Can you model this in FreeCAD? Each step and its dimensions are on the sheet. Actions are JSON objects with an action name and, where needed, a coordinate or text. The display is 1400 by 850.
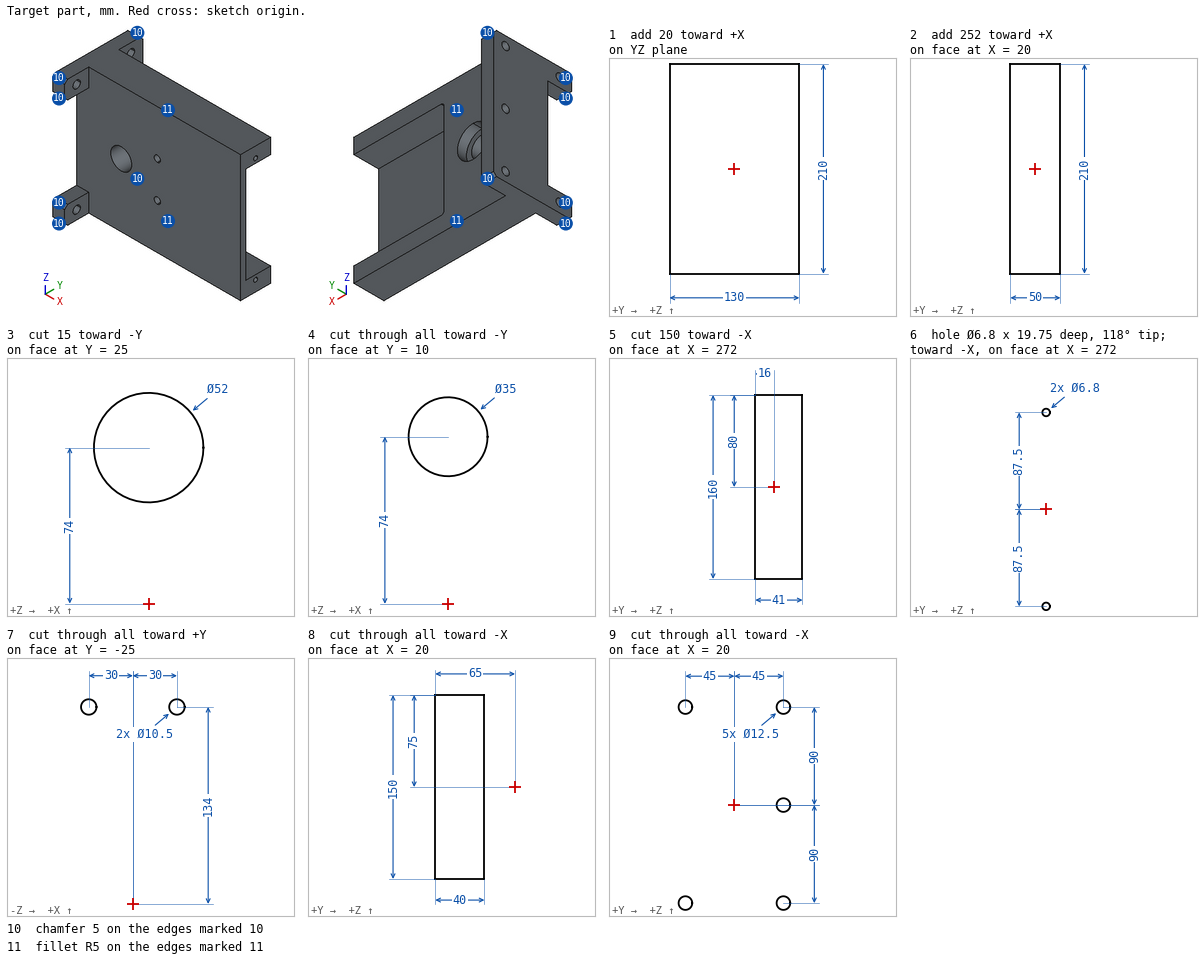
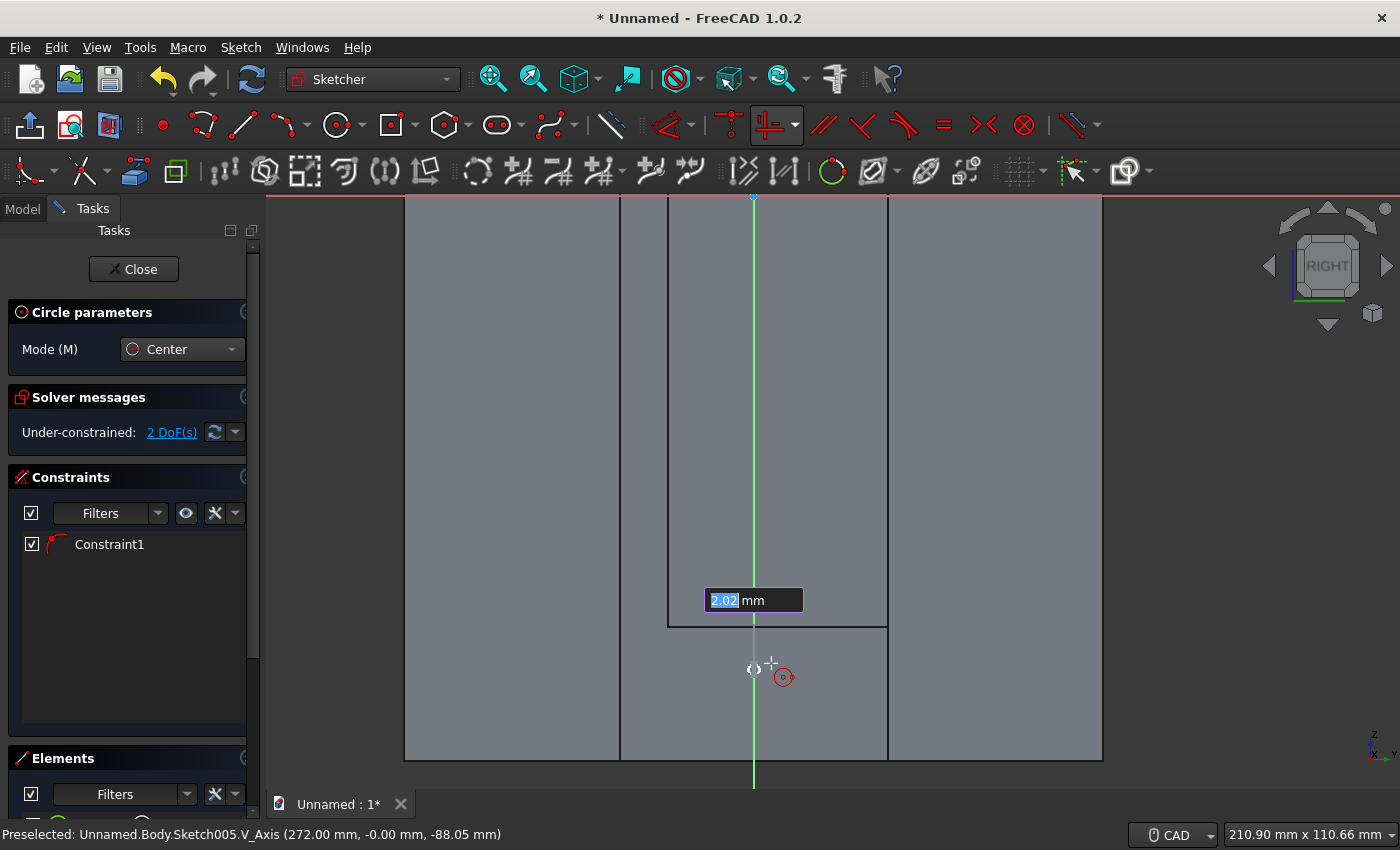
{"action": "left_click", "coordinate": [771, 661]}
{"action": "key", "text": "Escape"}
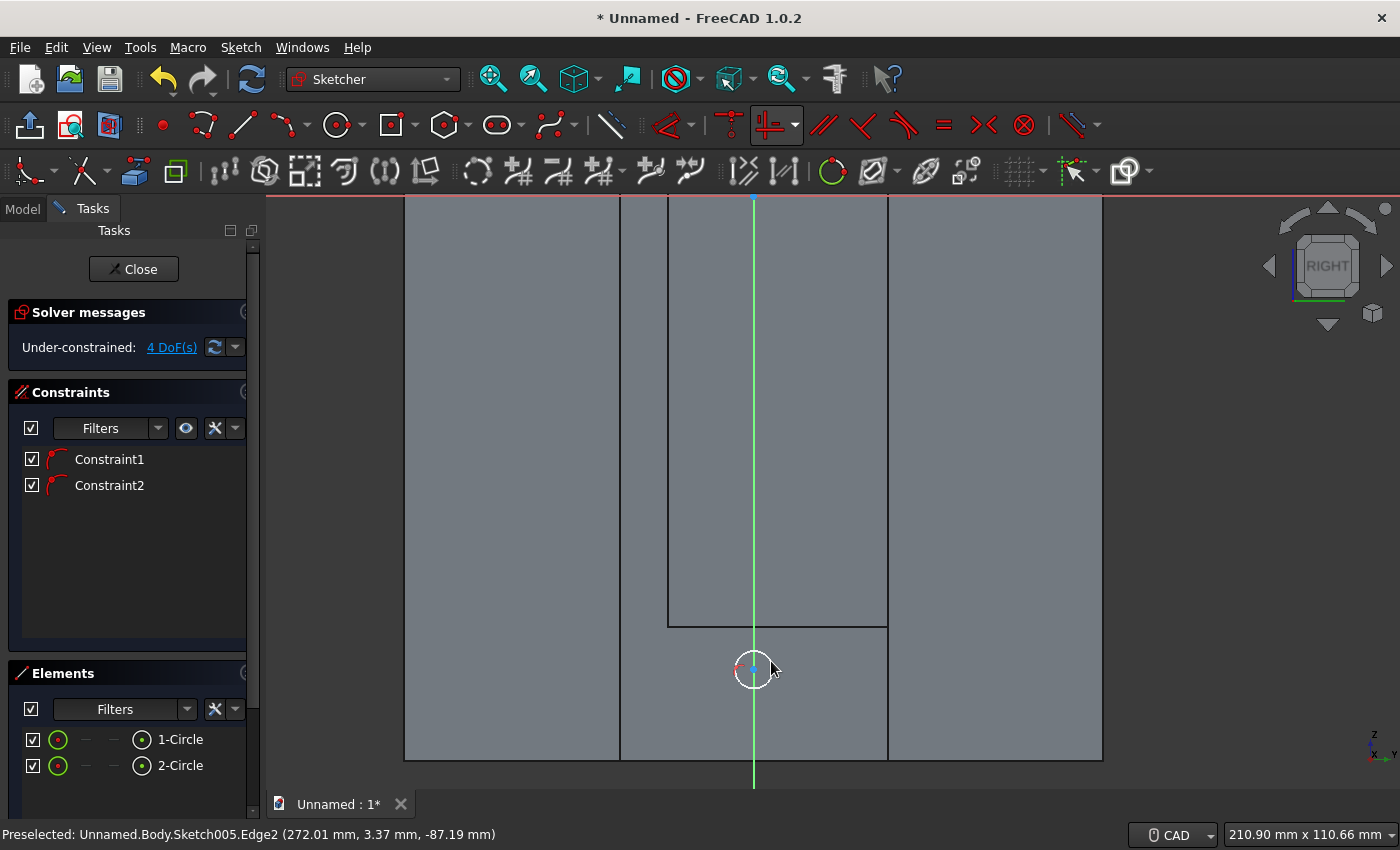
{"action": "scroll", "coordinate": [771, 663], "scroll_direction": "down", "scroll_amount": 5}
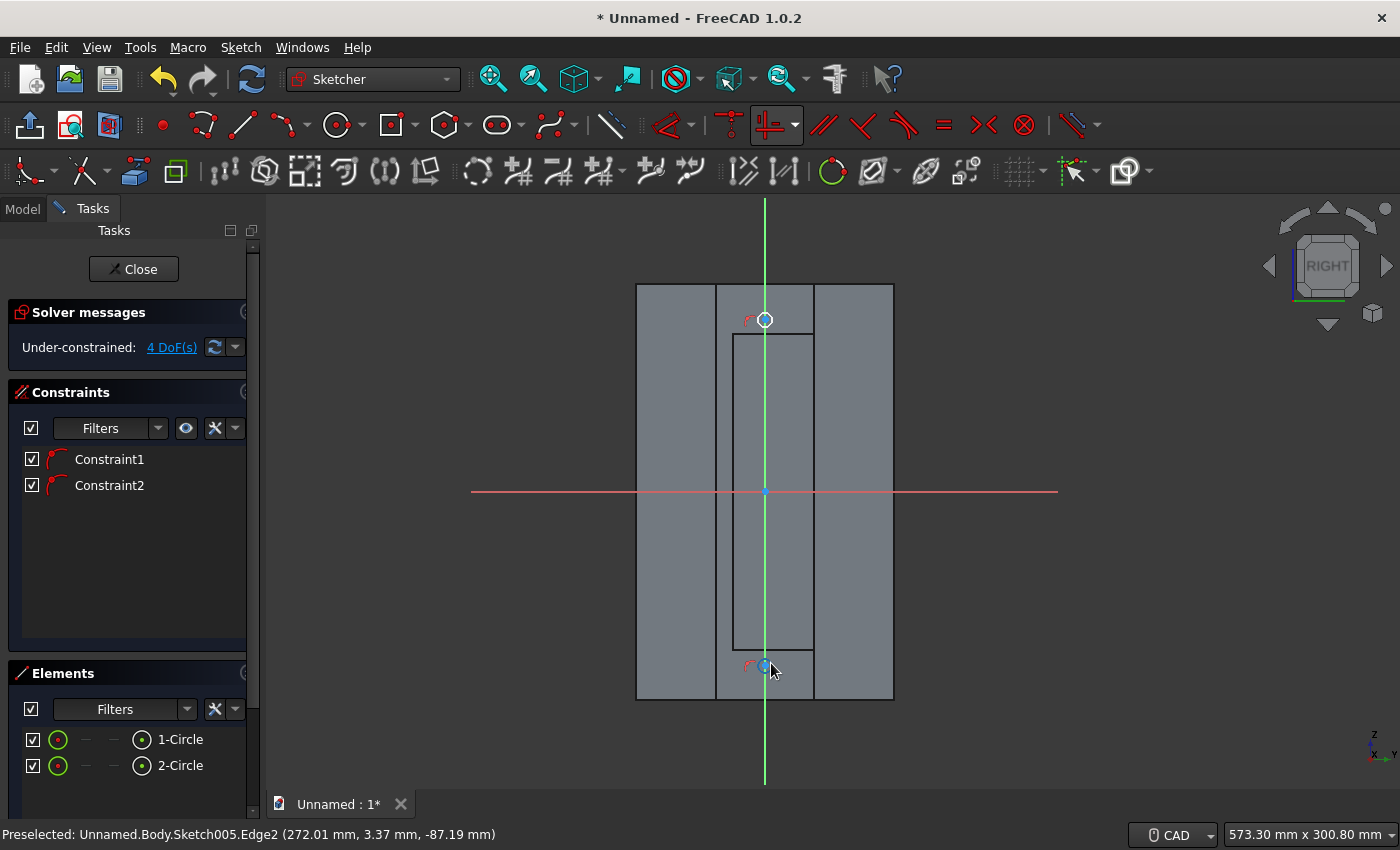
{"action": "scroll", "coordinate": [770, 315], "scroll_direction": "up", "scroll_amount": 6}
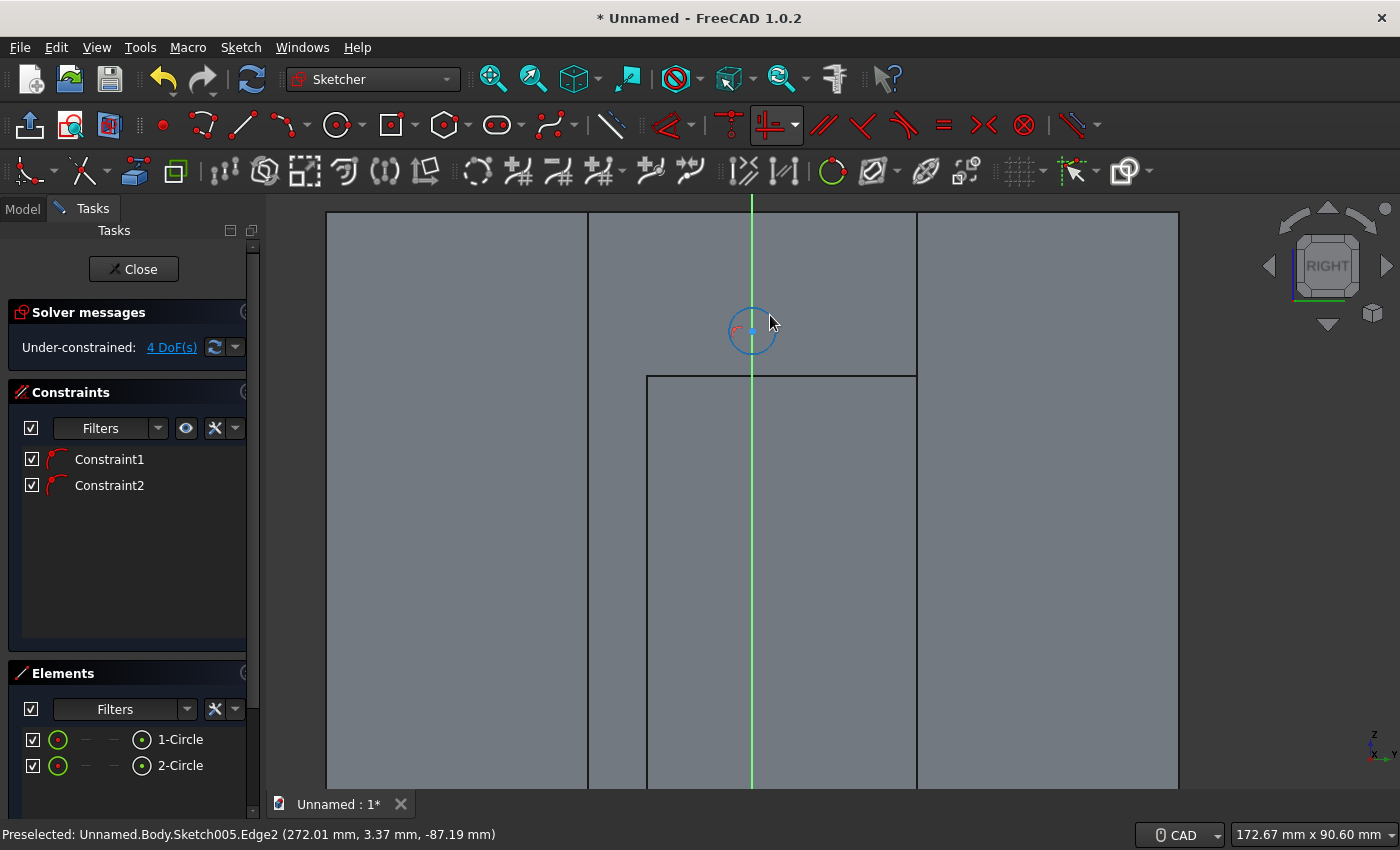
{"action": "left_click", "coordinate": [769, 315]}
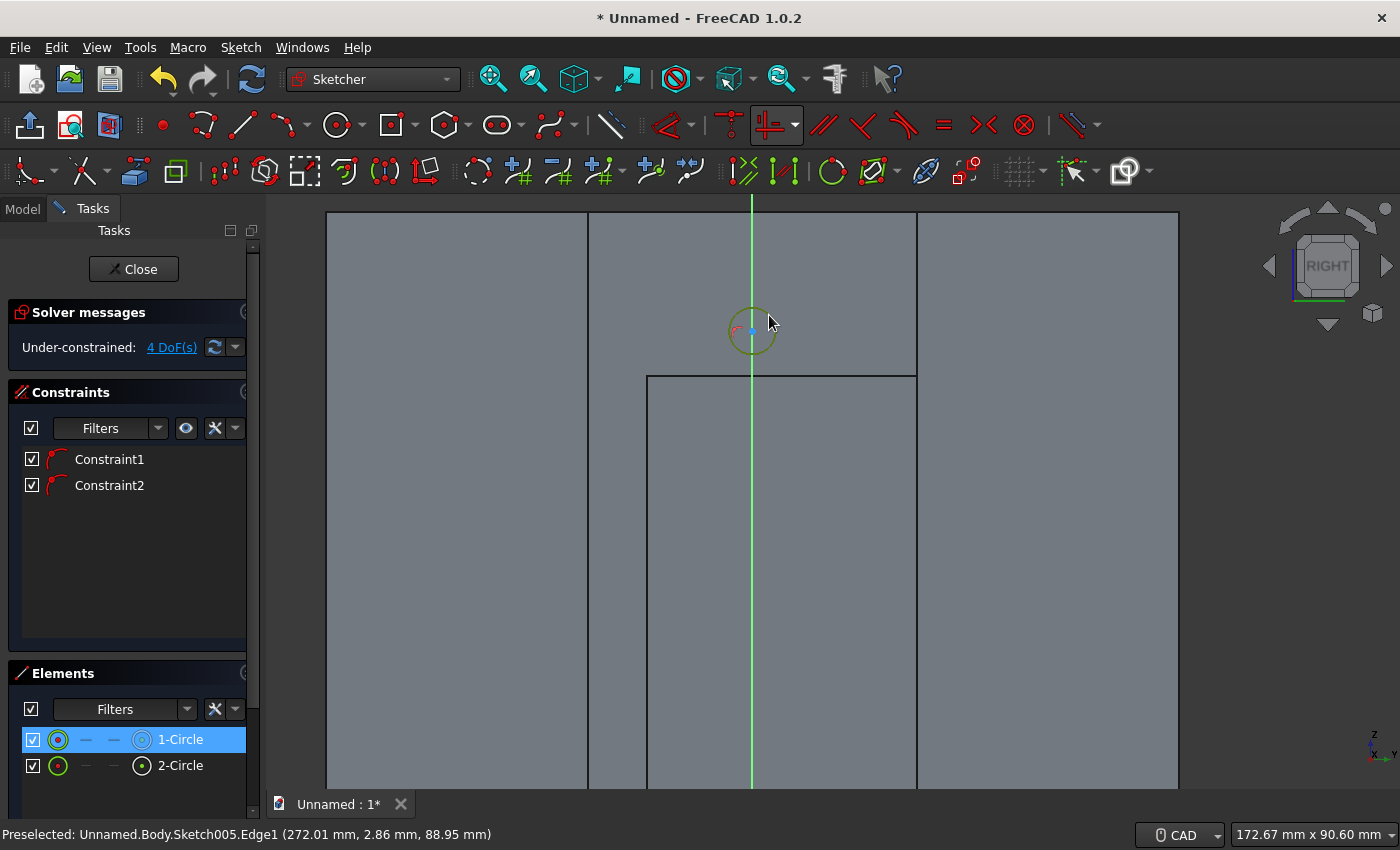
{"action": "scroll", "coordinate": [770, 315], "scroll_direction": "down", "scroll_amount": 6}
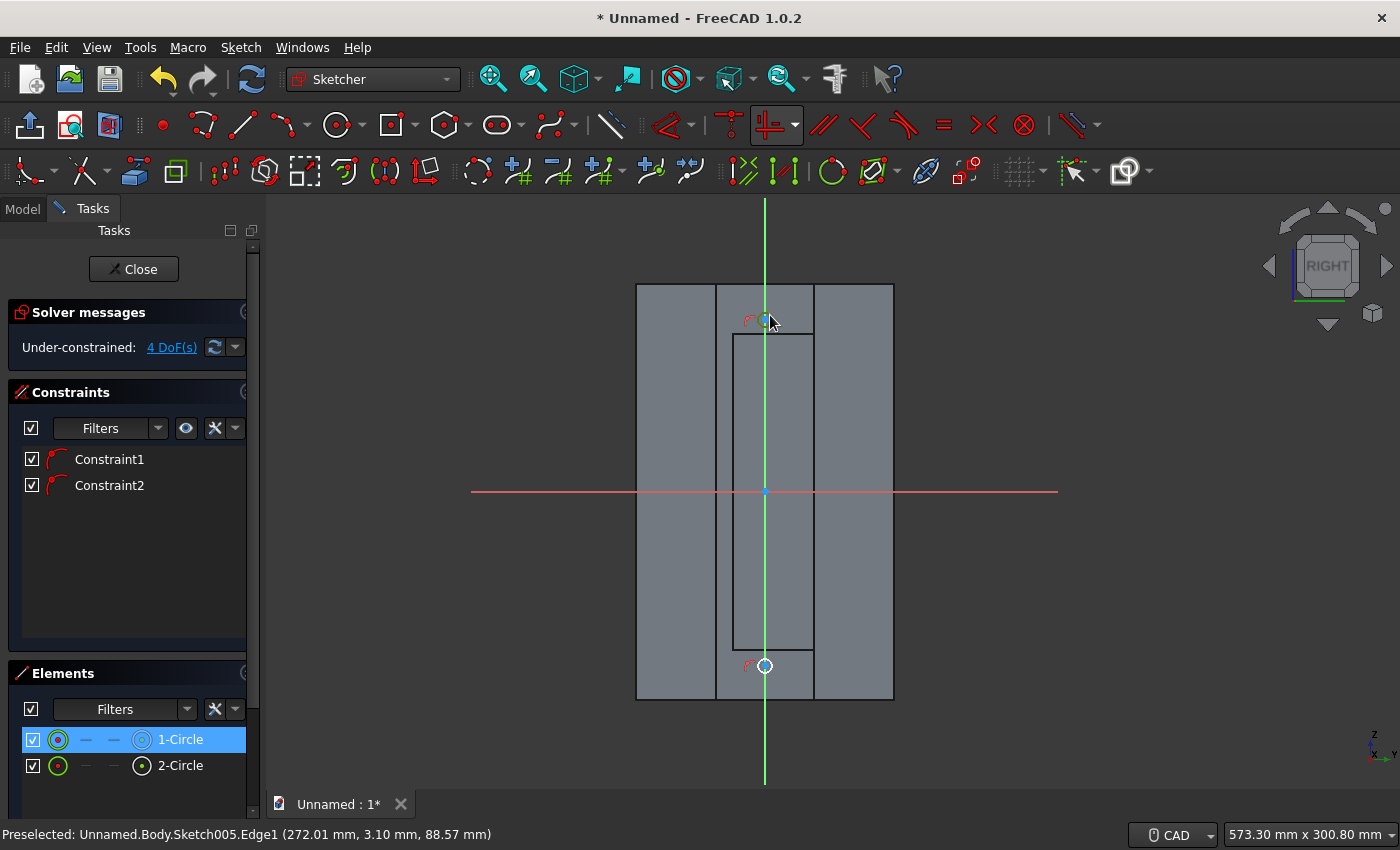
{"action": "scroll", "coordinate": [770, 661], "scroll_direction": "up", "scroll_amount": 6}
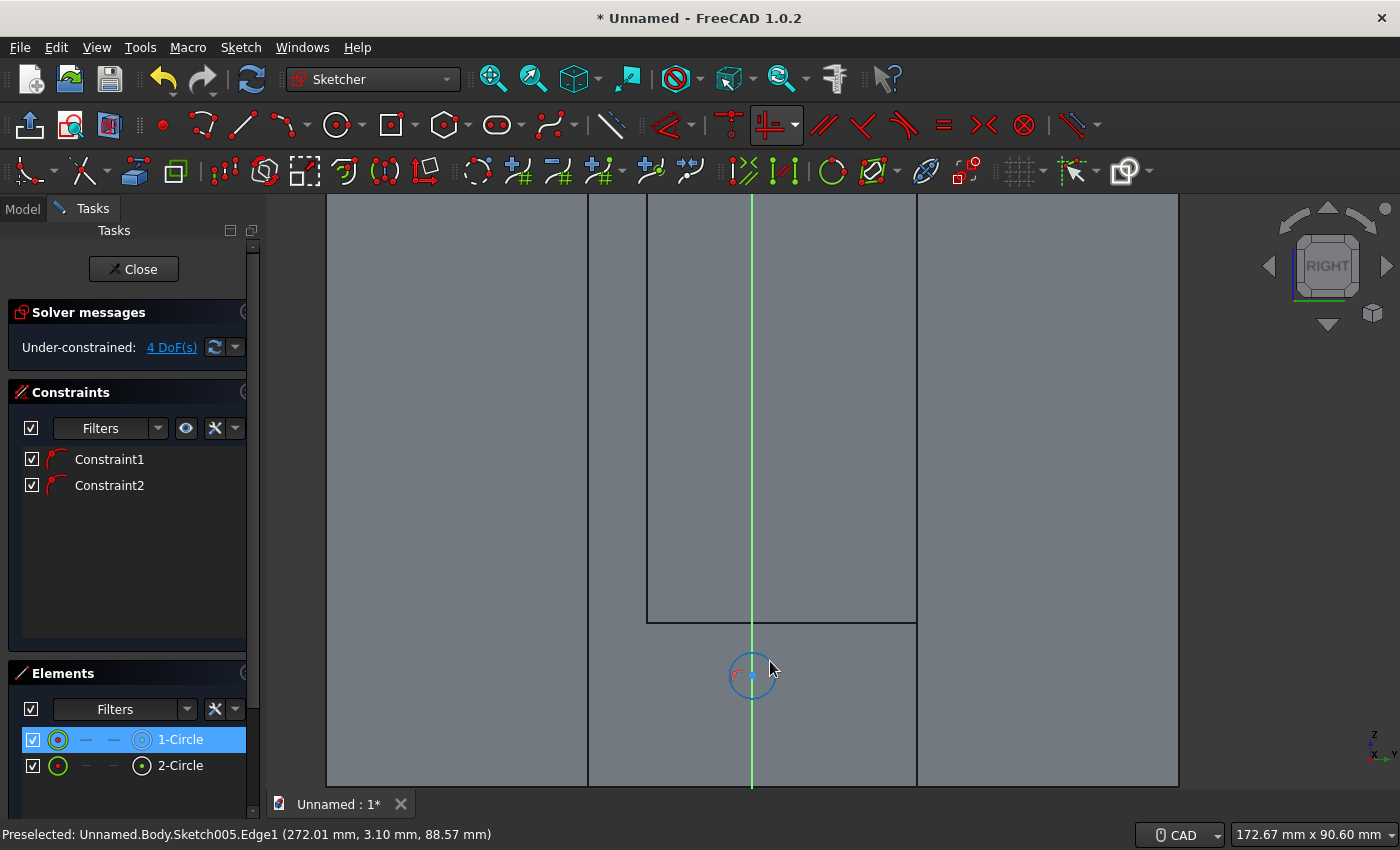
{"action": "left_click", "coordinate": [769, 660]}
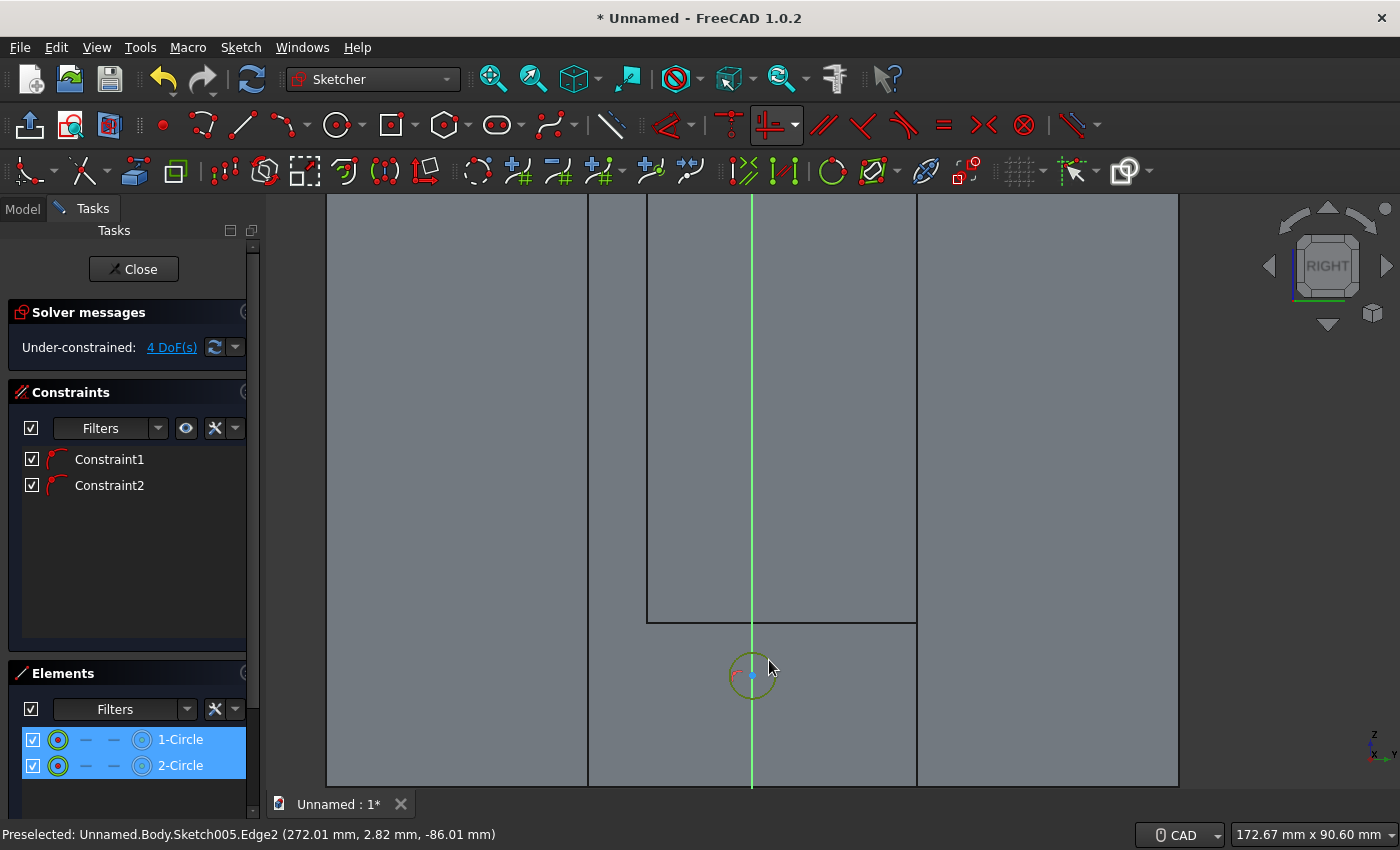
{"action": "left_click", "coordinate": [944, 126]}